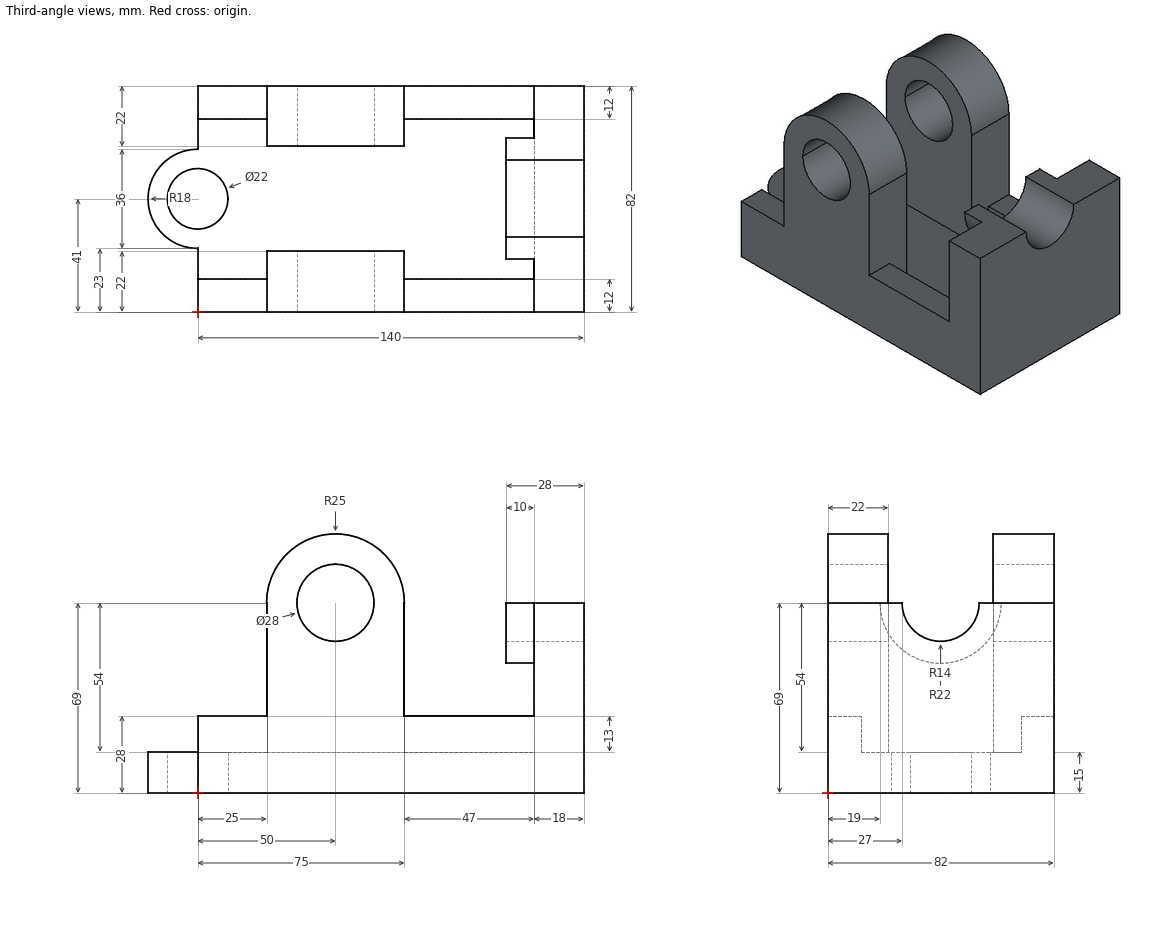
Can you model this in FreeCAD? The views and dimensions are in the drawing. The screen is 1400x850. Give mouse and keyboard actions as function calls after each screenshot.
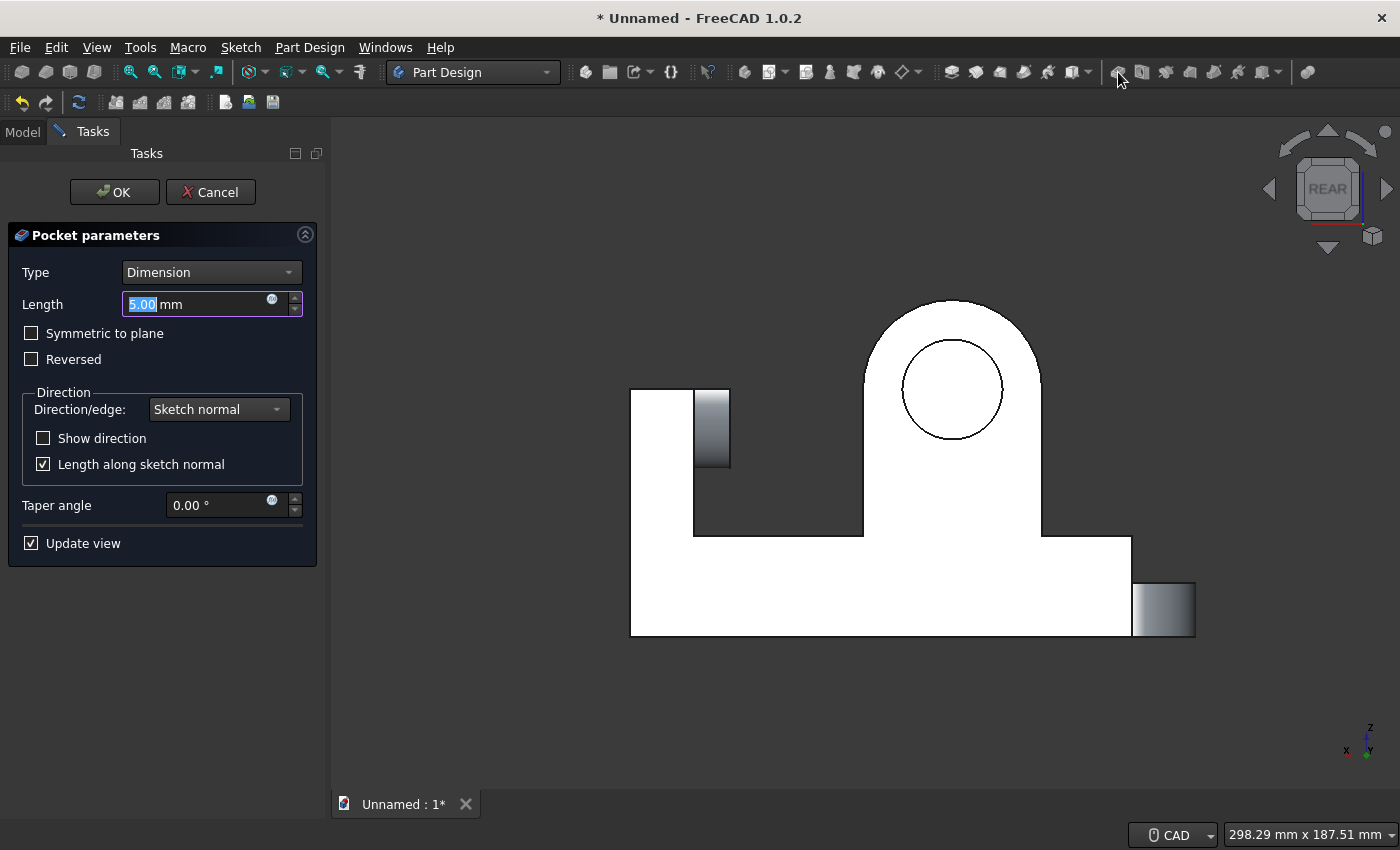
text(22)
key(Tab)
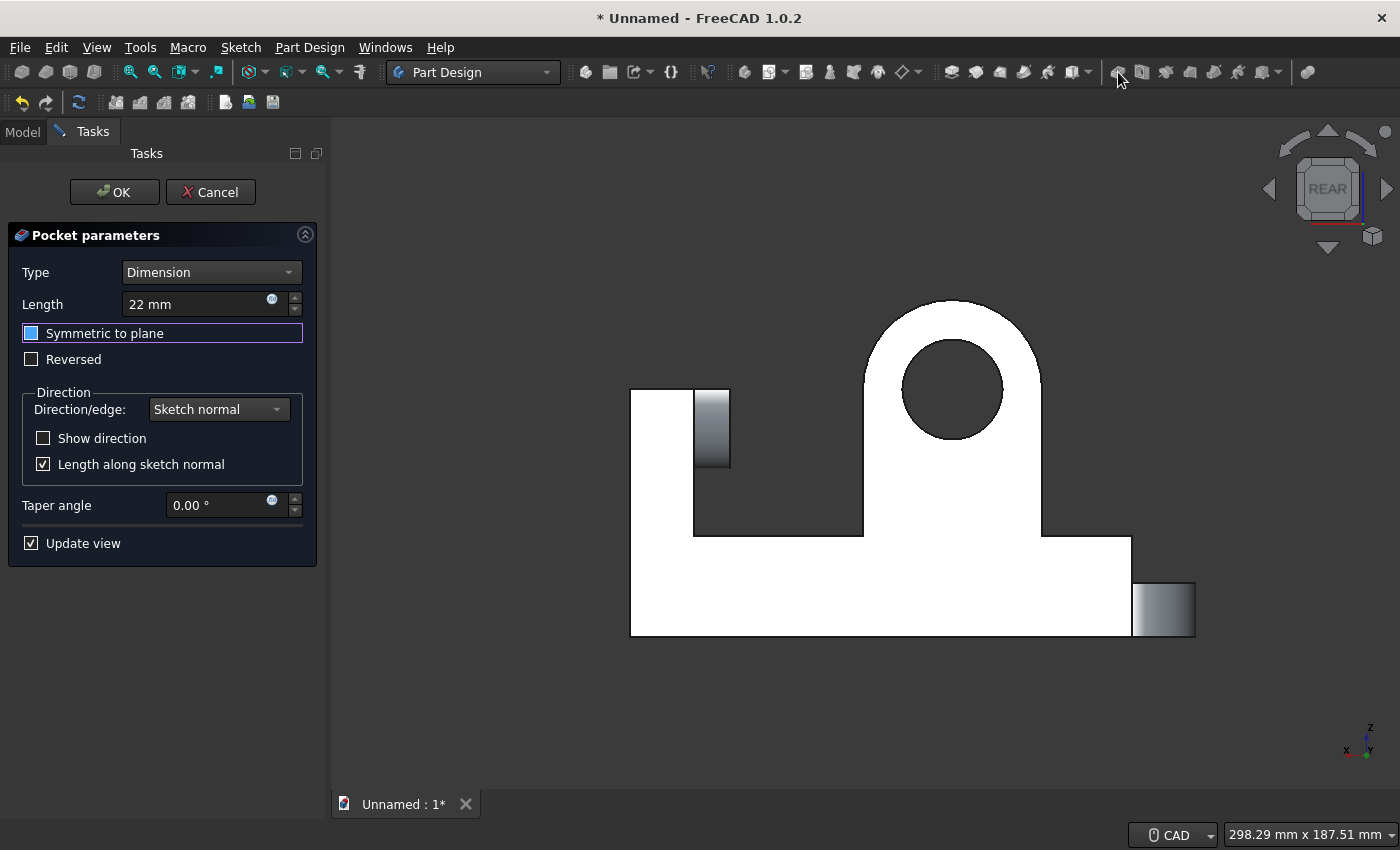
click(115, 192)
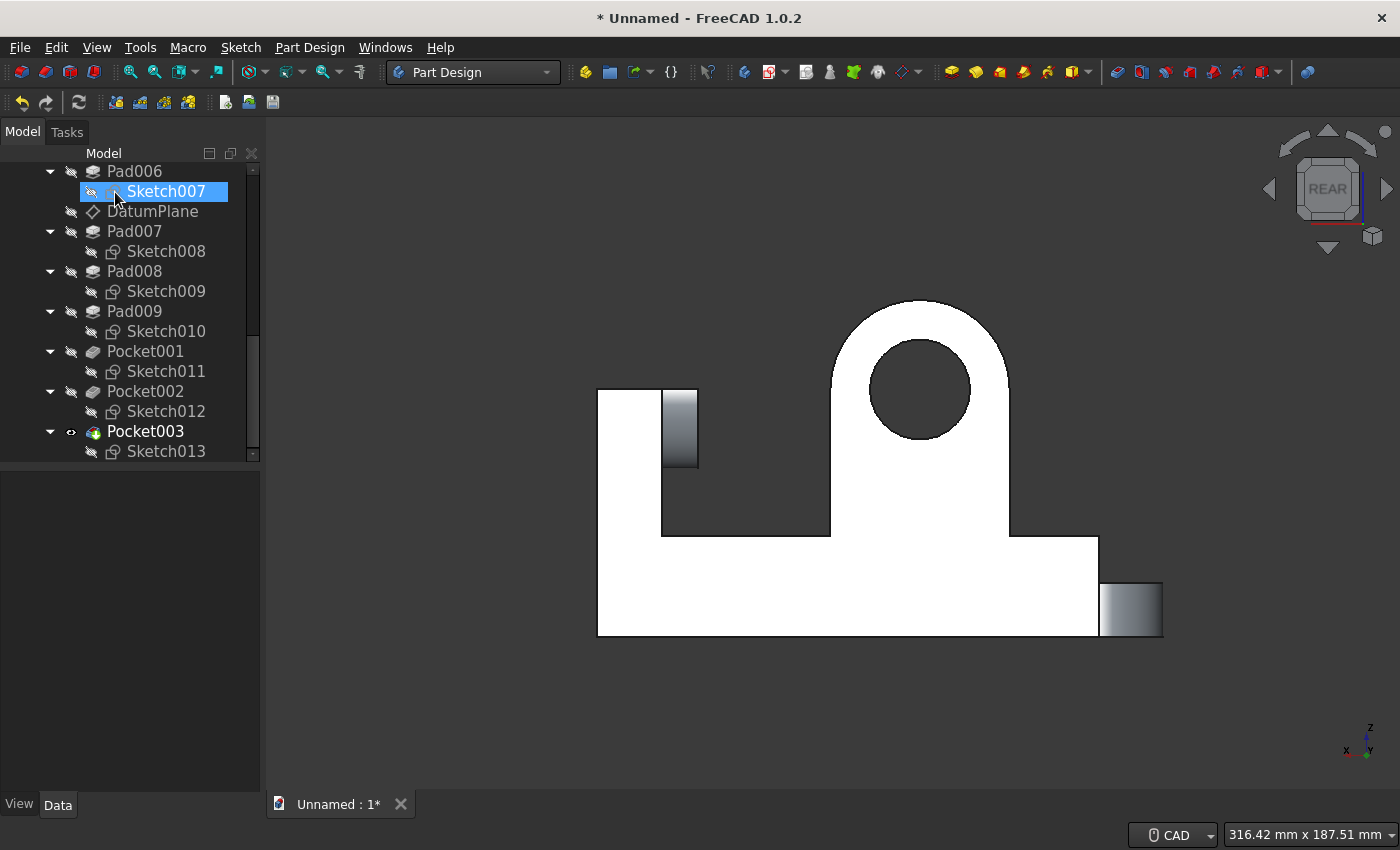
key(0)